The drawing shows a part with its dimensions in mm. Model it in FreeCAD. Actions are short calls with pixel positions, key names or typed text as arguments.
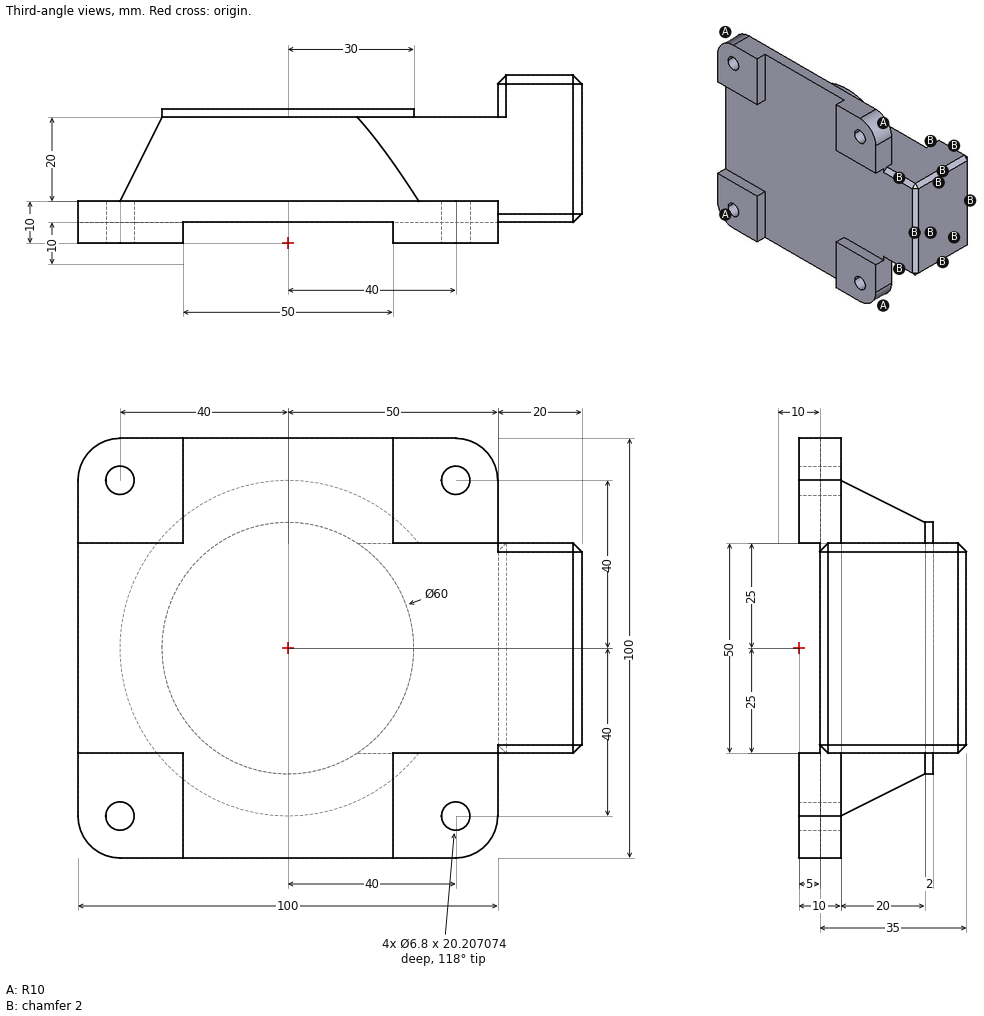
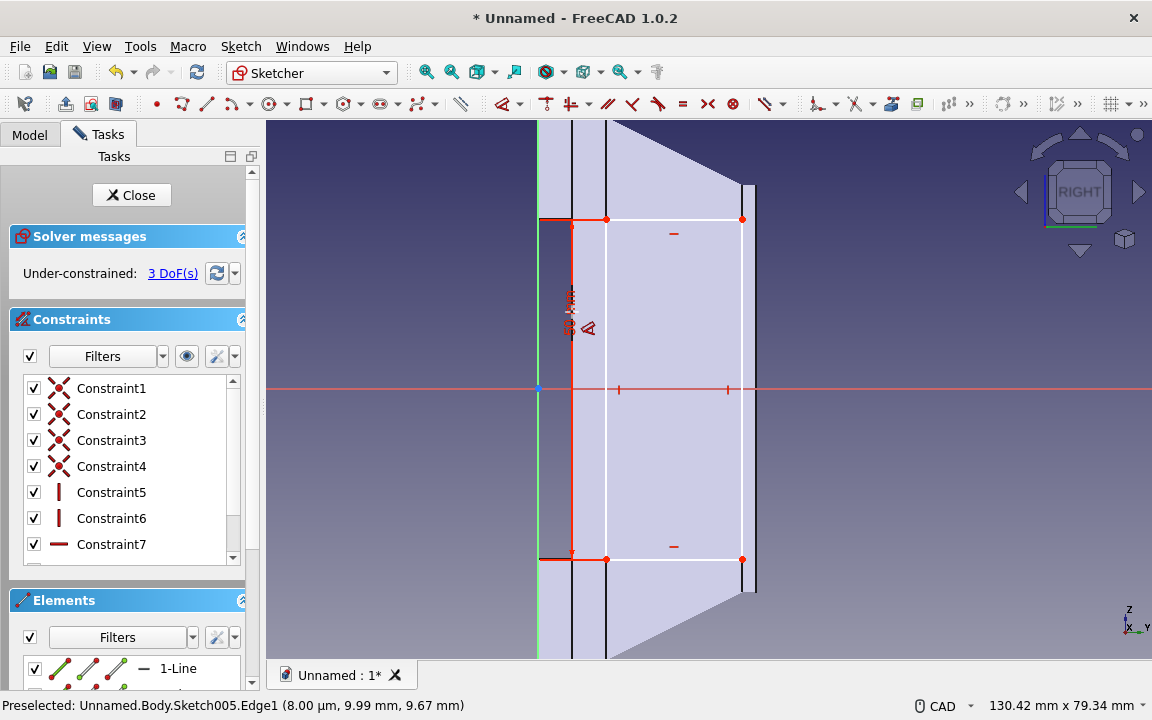
click(647, 560)
click(674, 594)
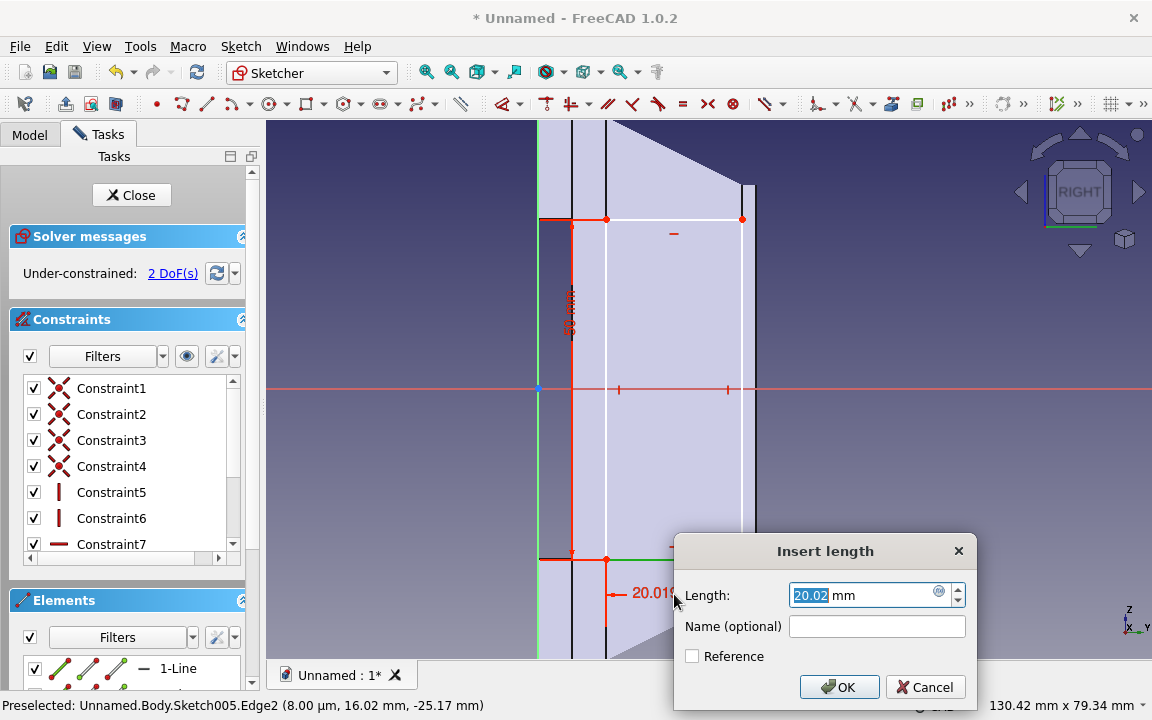
text(20)
key(Return)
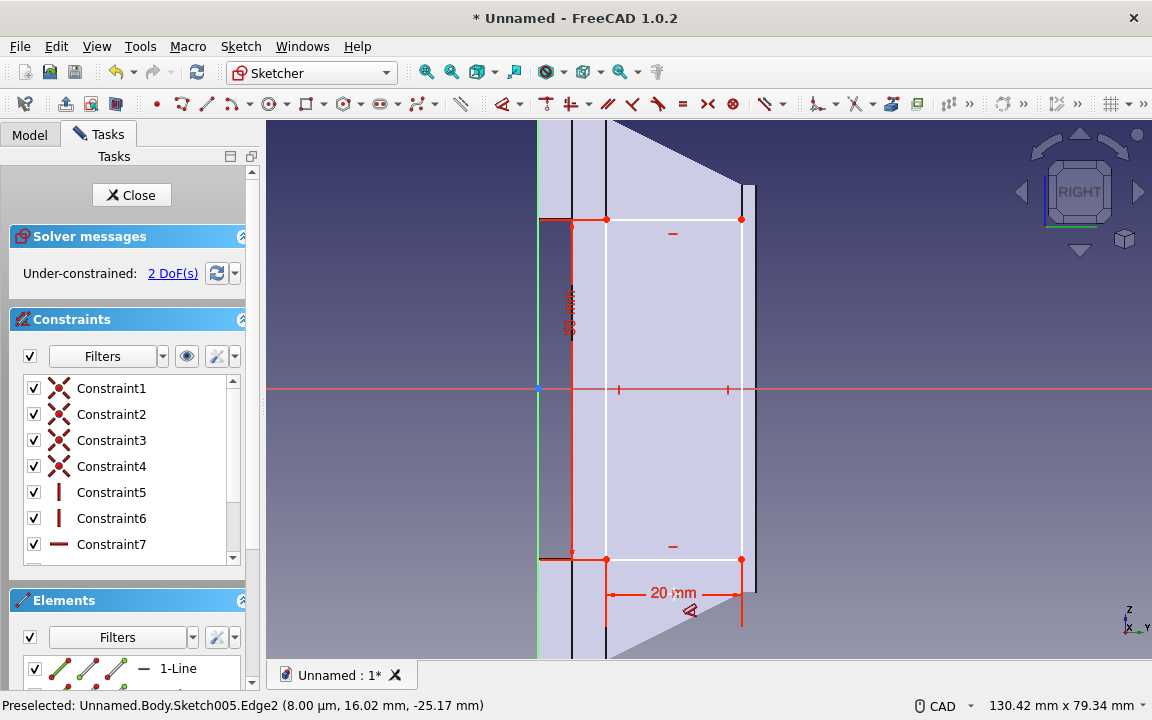
click(606, 220)
click(572, 186)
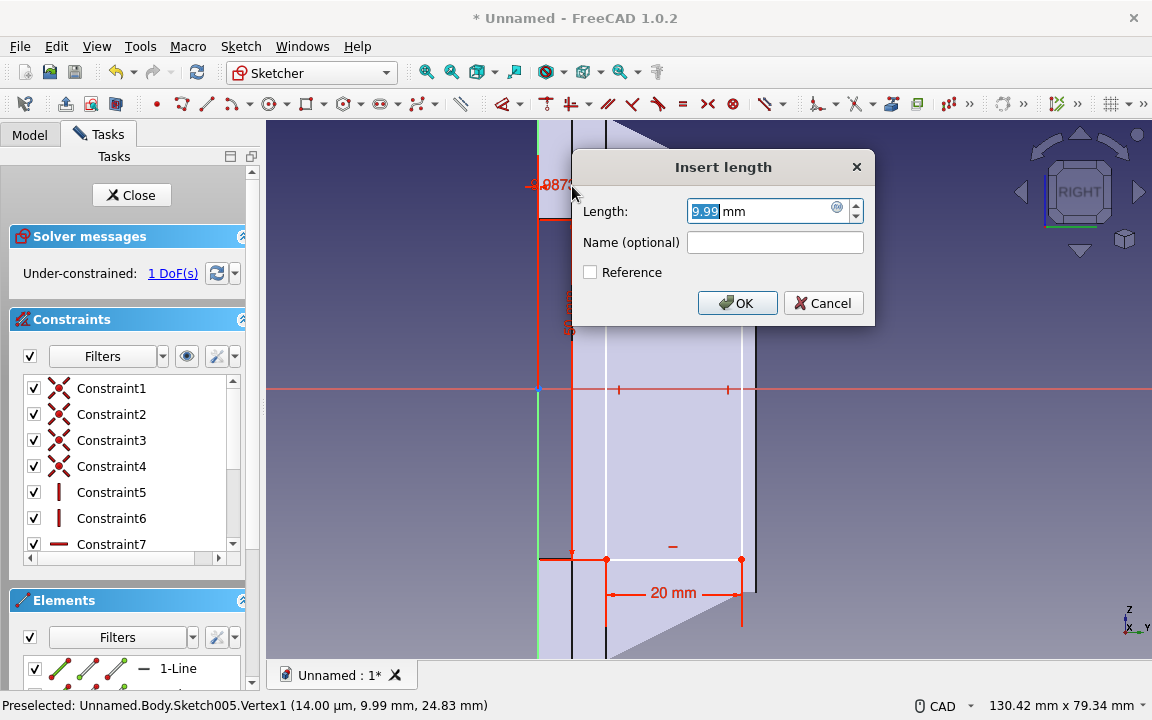
text(10)
key(Return)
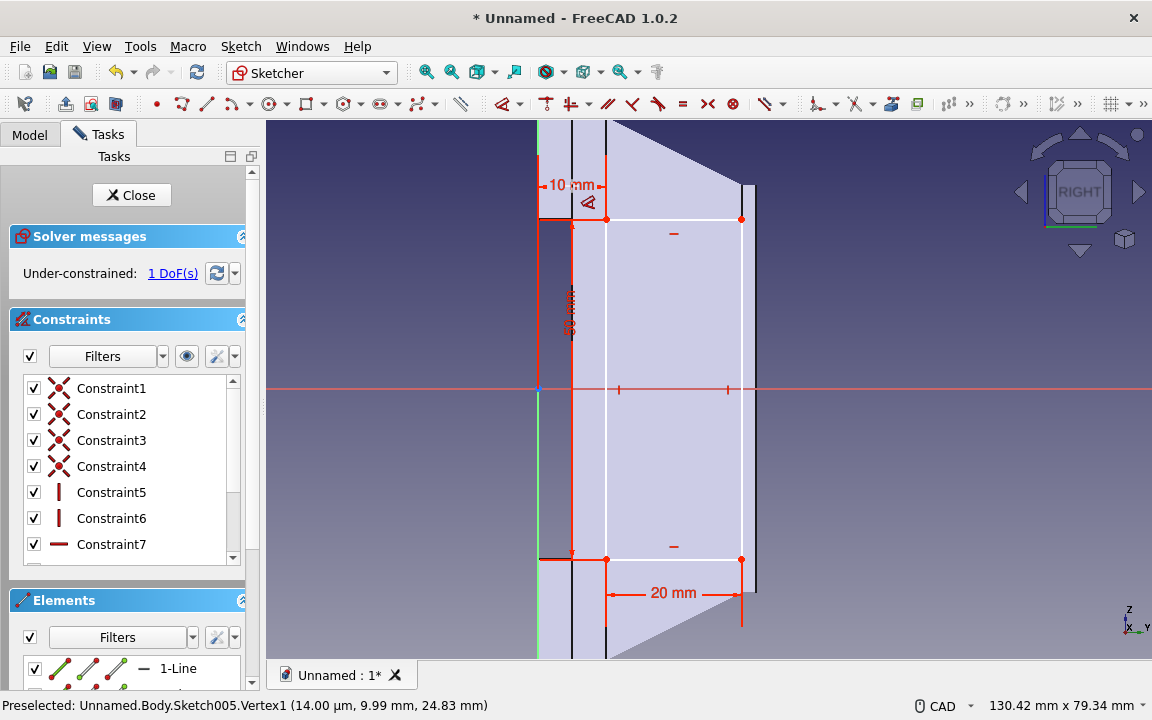
click(606, 220)
click(504, 266)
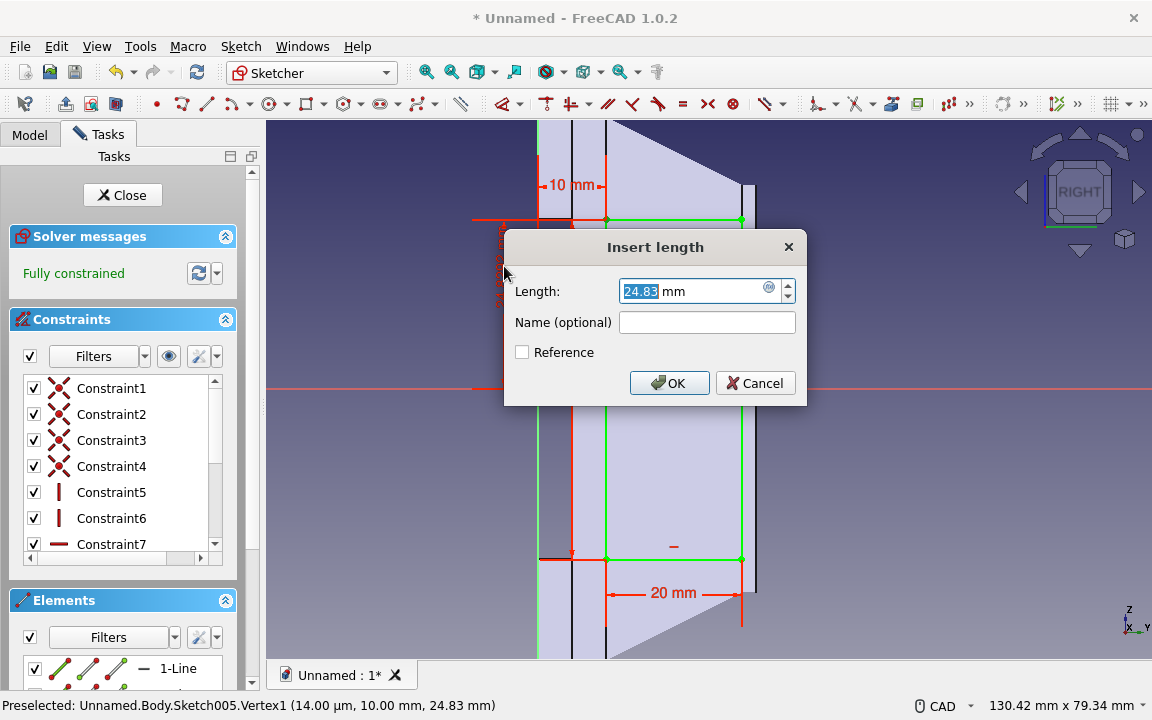
text(25)
key(Return)
key(Escape)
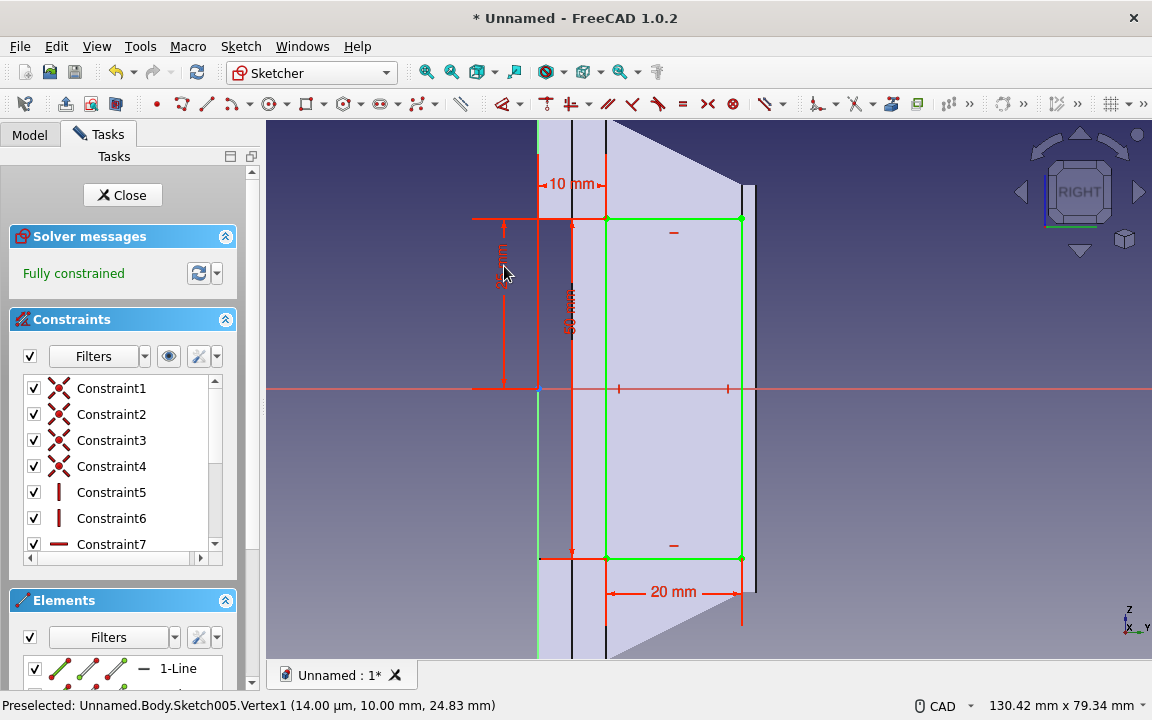
click(123, 195)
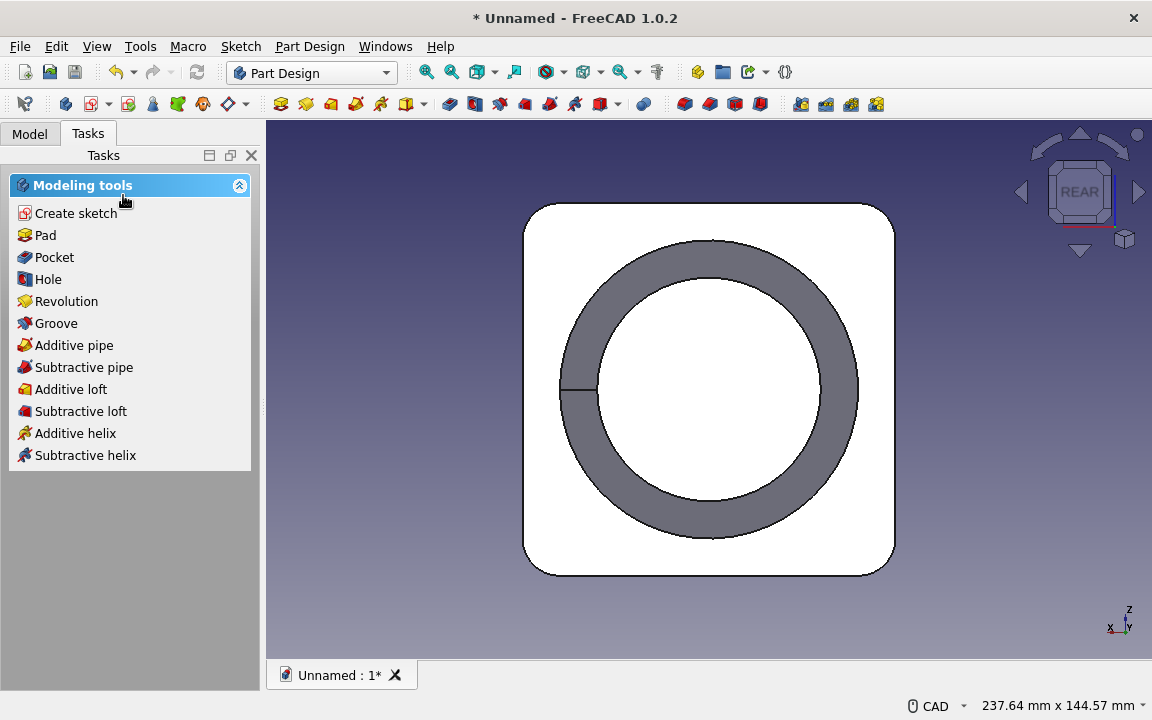
click(281, 104)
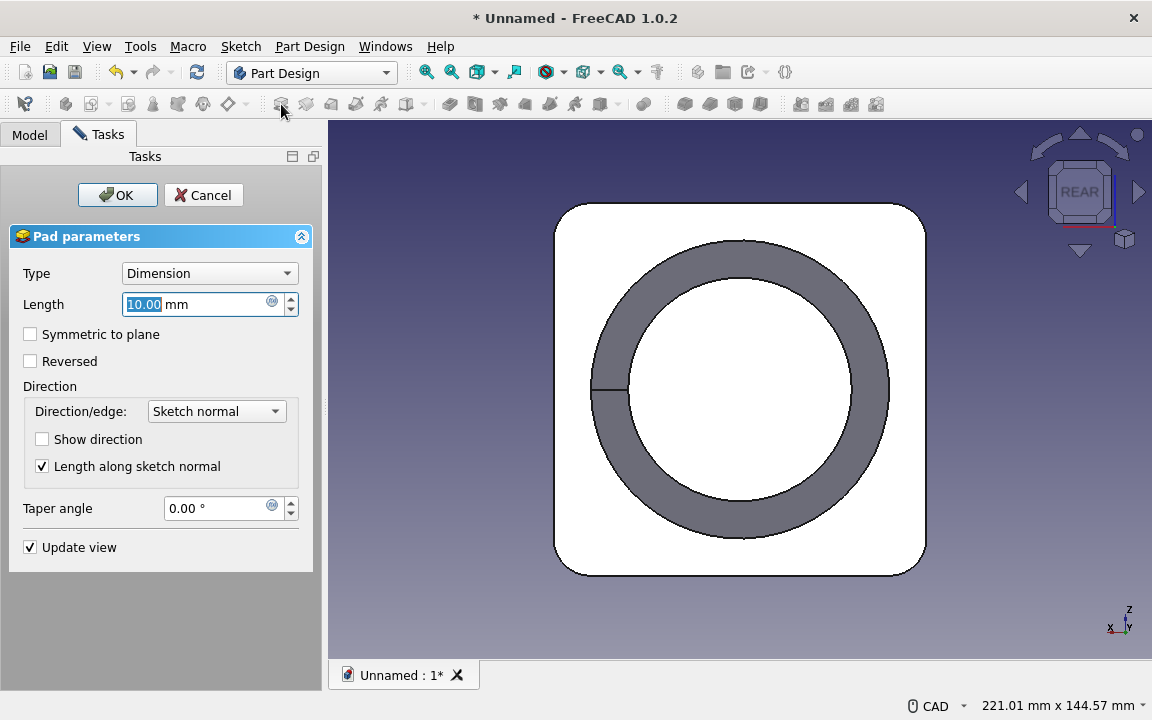
text(50)
key(Tab)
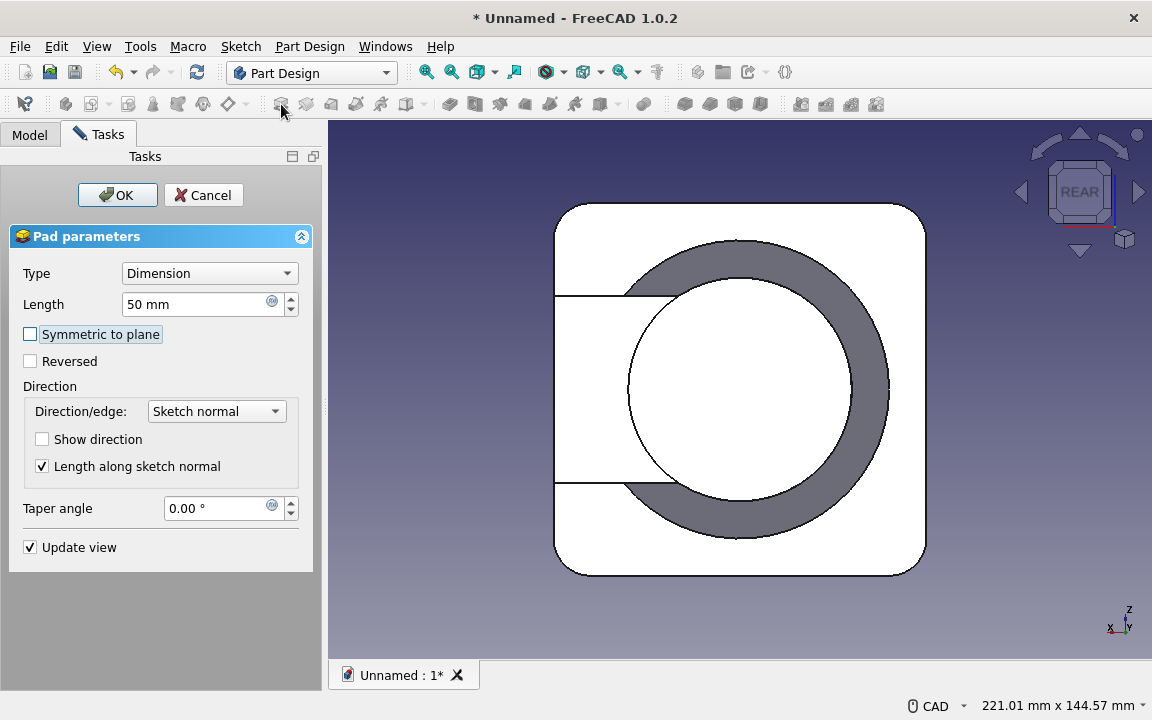
click(118, 195)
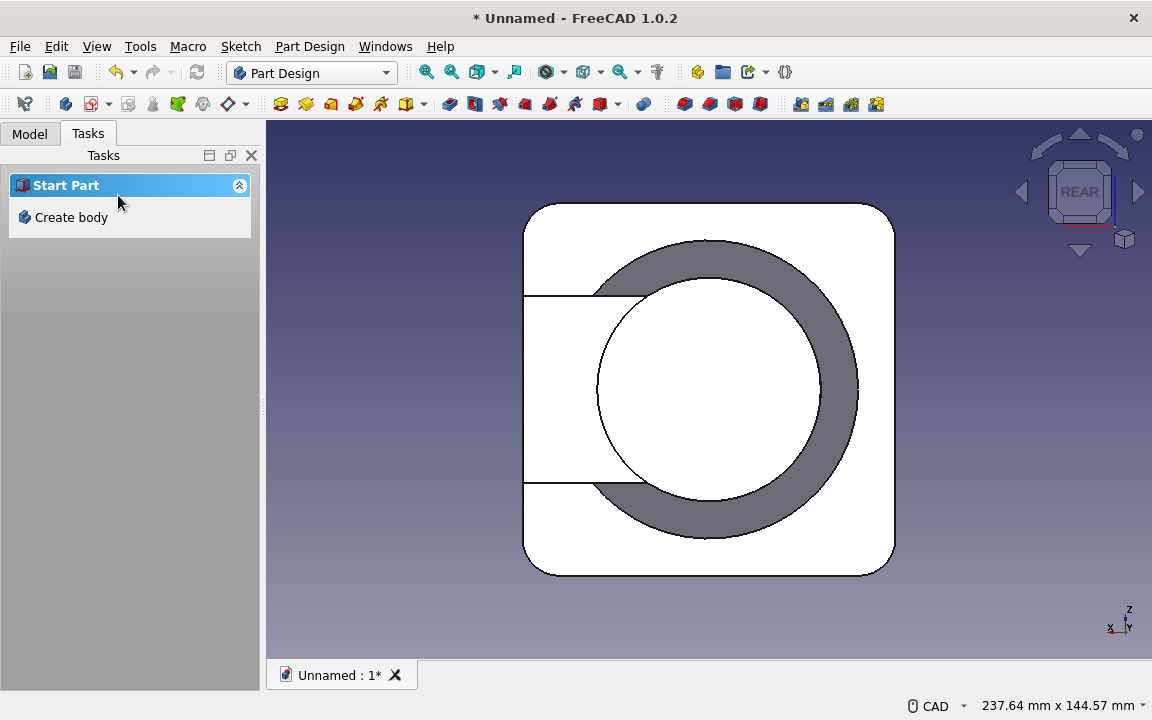
key(0)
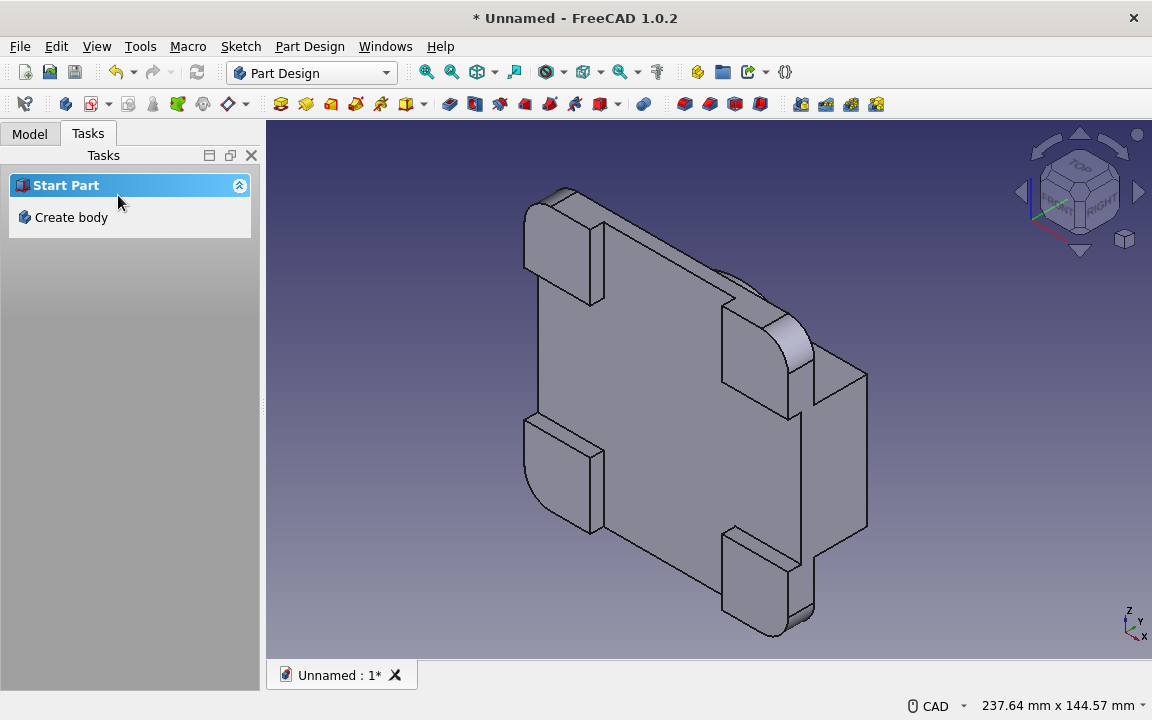
click(839, 431)